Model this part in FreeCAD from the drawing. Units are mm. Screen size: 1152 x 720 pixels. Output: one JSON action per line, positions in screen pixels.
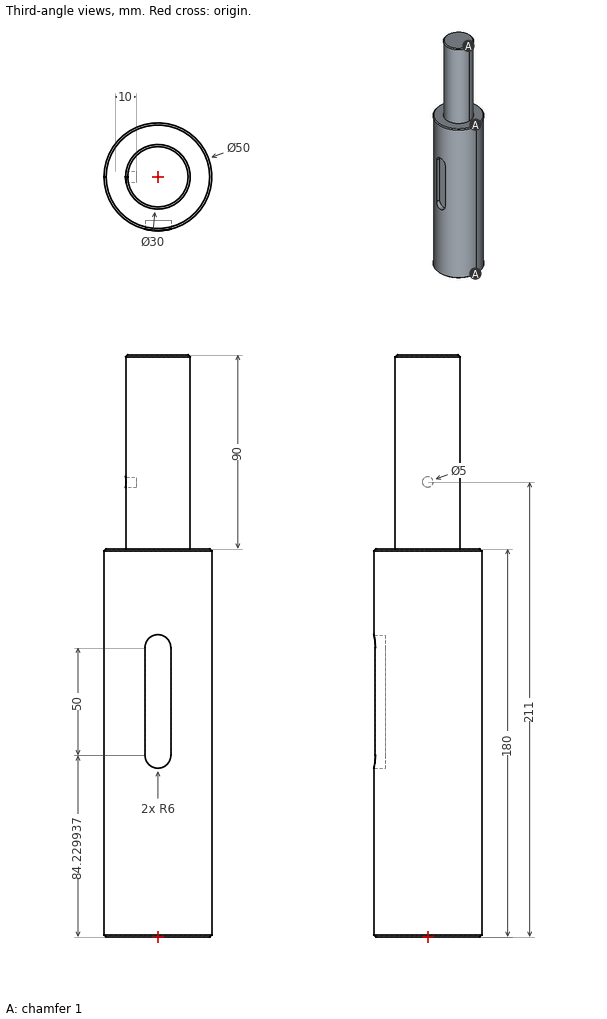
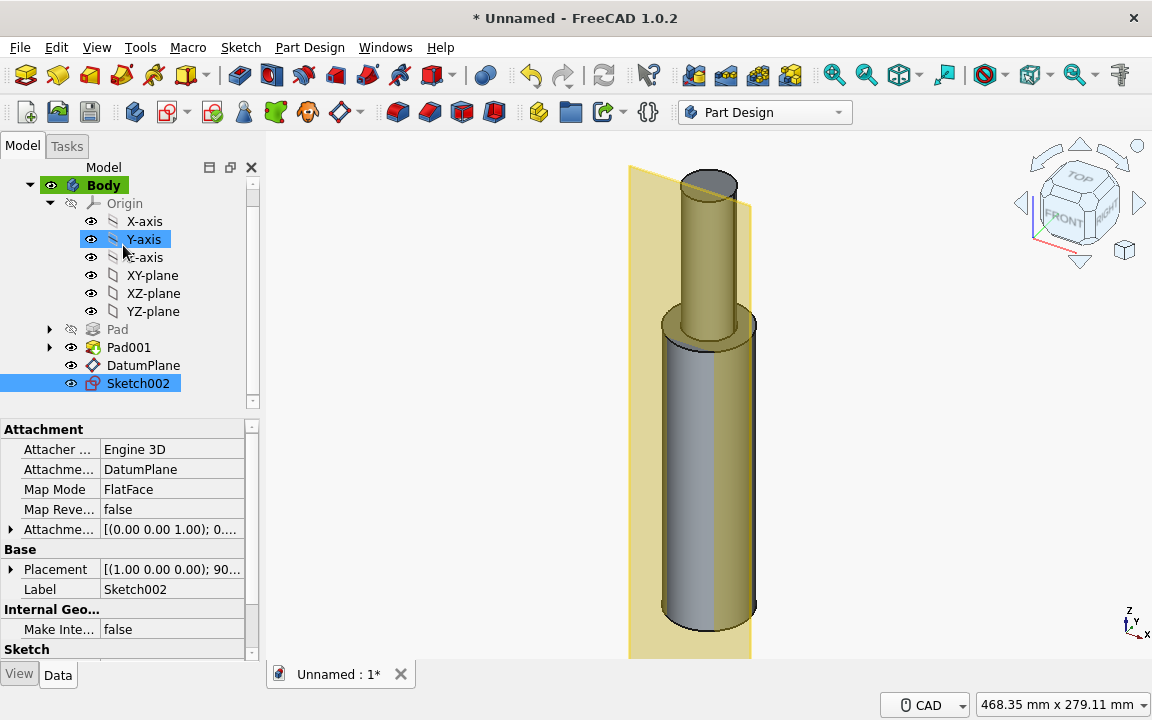
{"action": "left_click", "coordinate": [240, 76]}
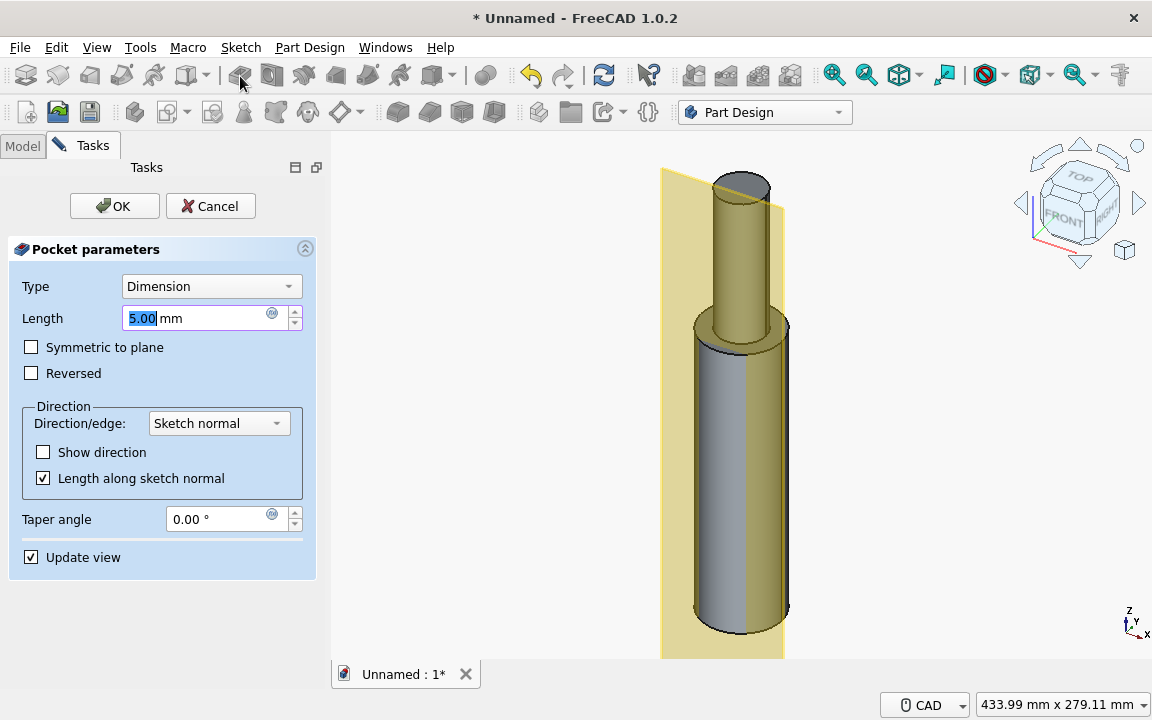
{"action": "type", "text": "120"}
{"action": "key", "text": "Tab"}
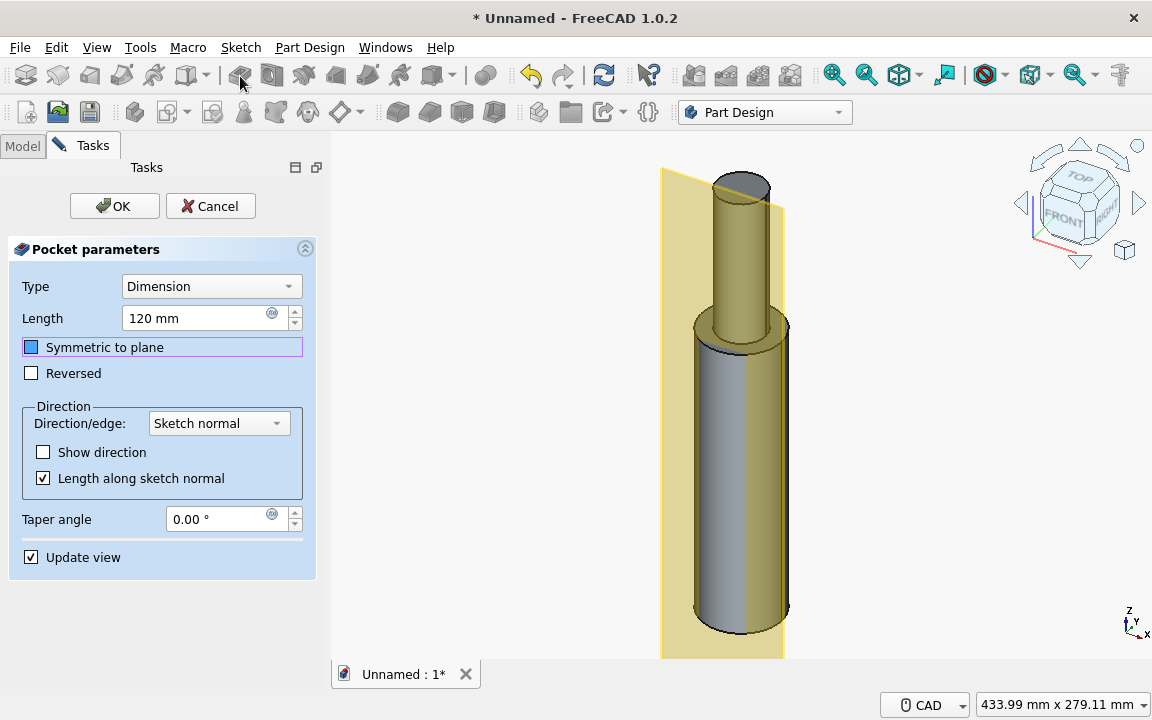
{"action": "left_click", "coordinate": [30, 373]}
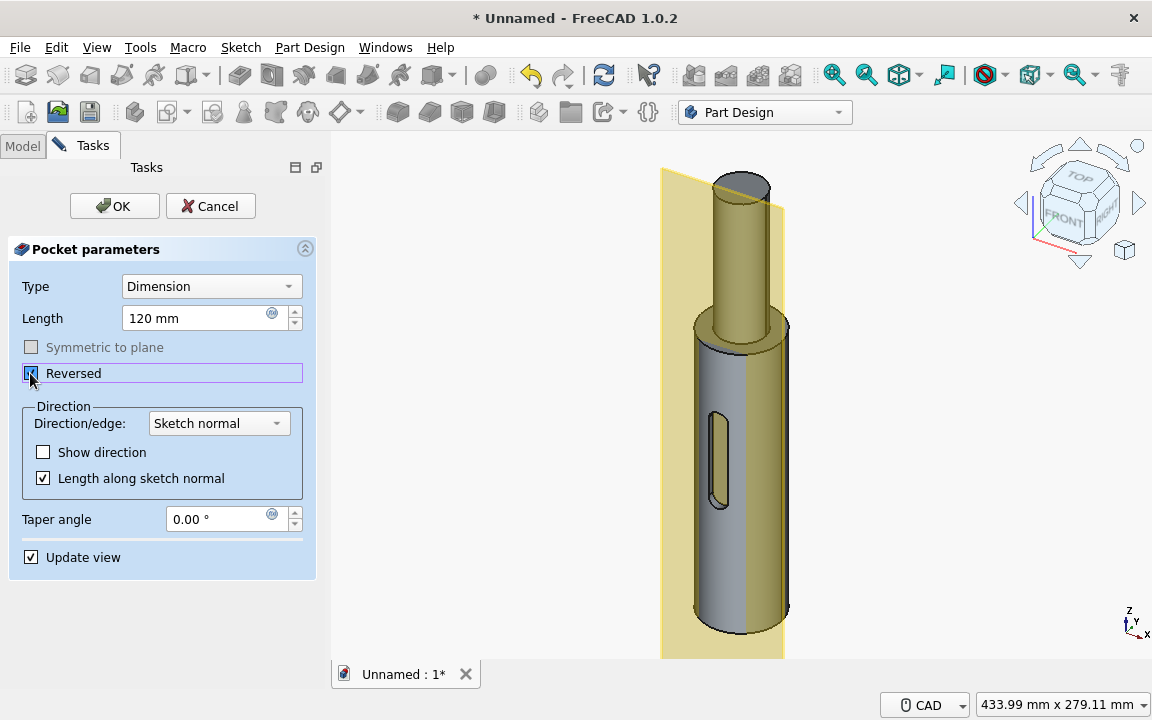
{"action": "left_click", "coordinate": [115, 206]}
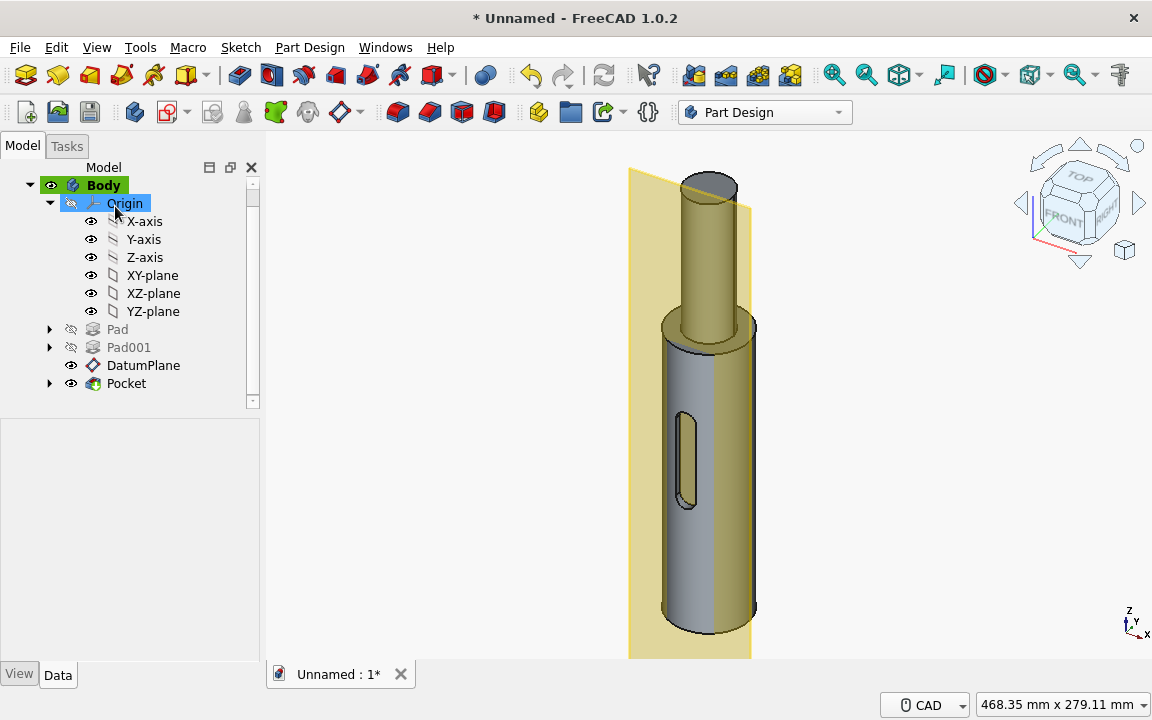
{"action": "left_click", "coordinate": [116, 365]}
{"action": "key", "text": "space"}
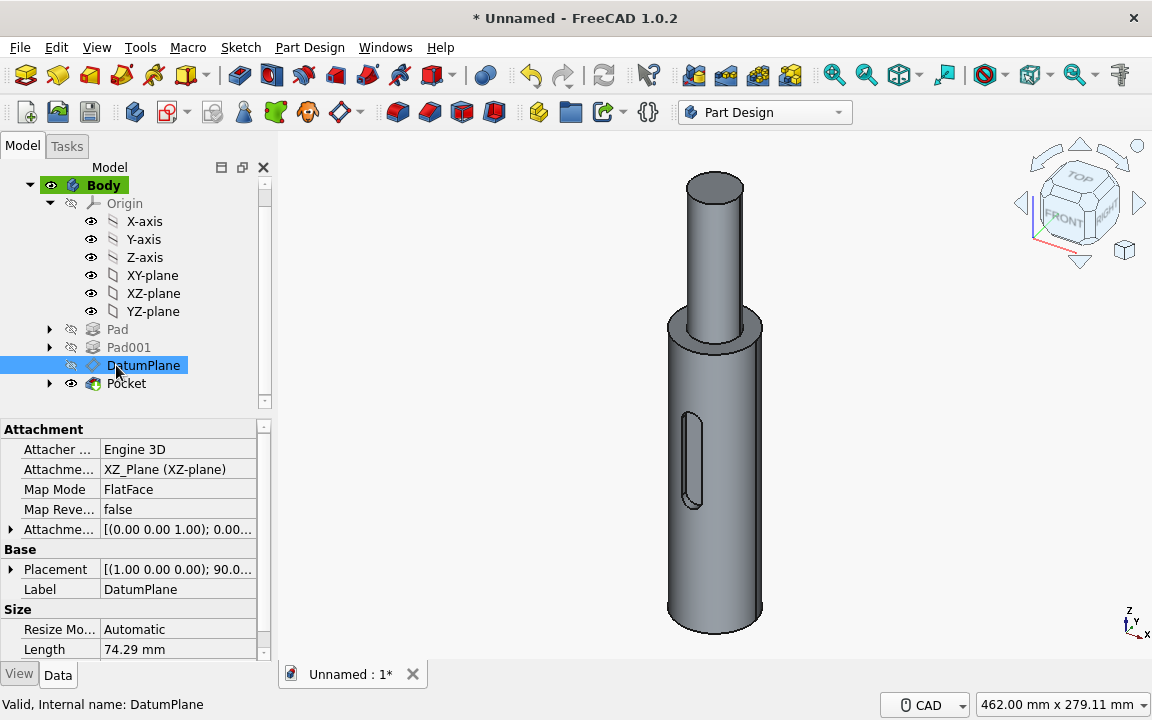
{"action": "left_click", "coordinate": [668, 330]}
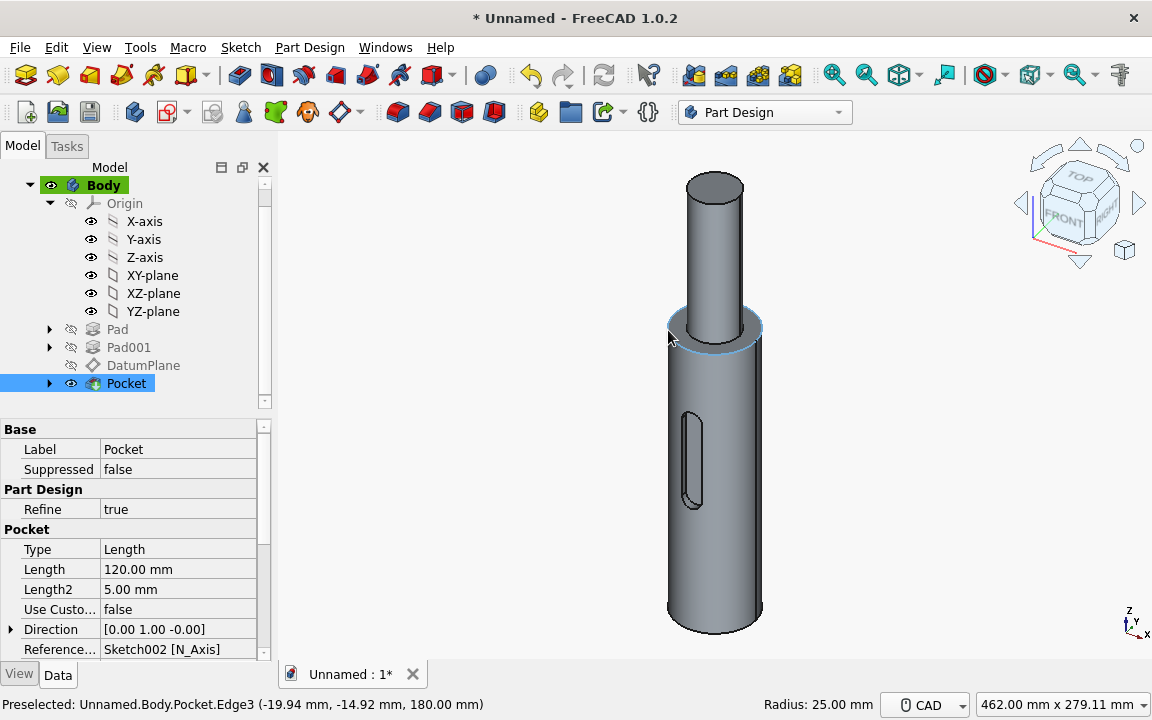
{"action": "left_click", "coordinate": [703, 172], "text": "ctrl"}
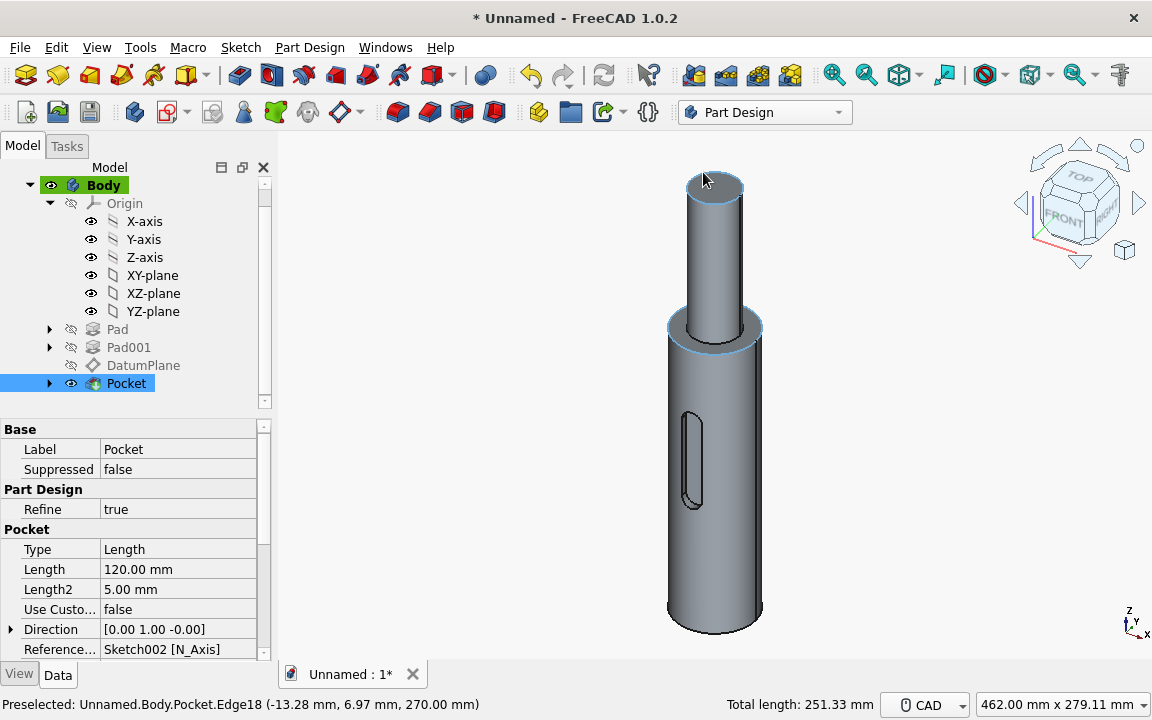
{"action": "key", "text": "0"}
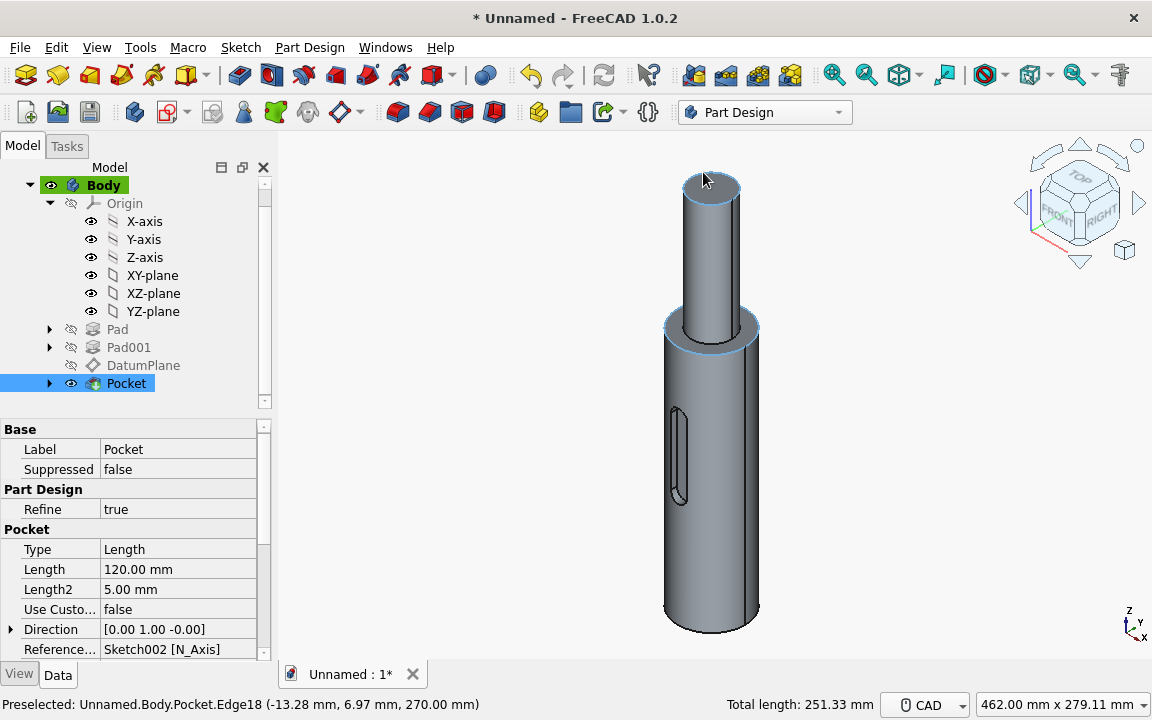
{"action": "key", "text": "2"}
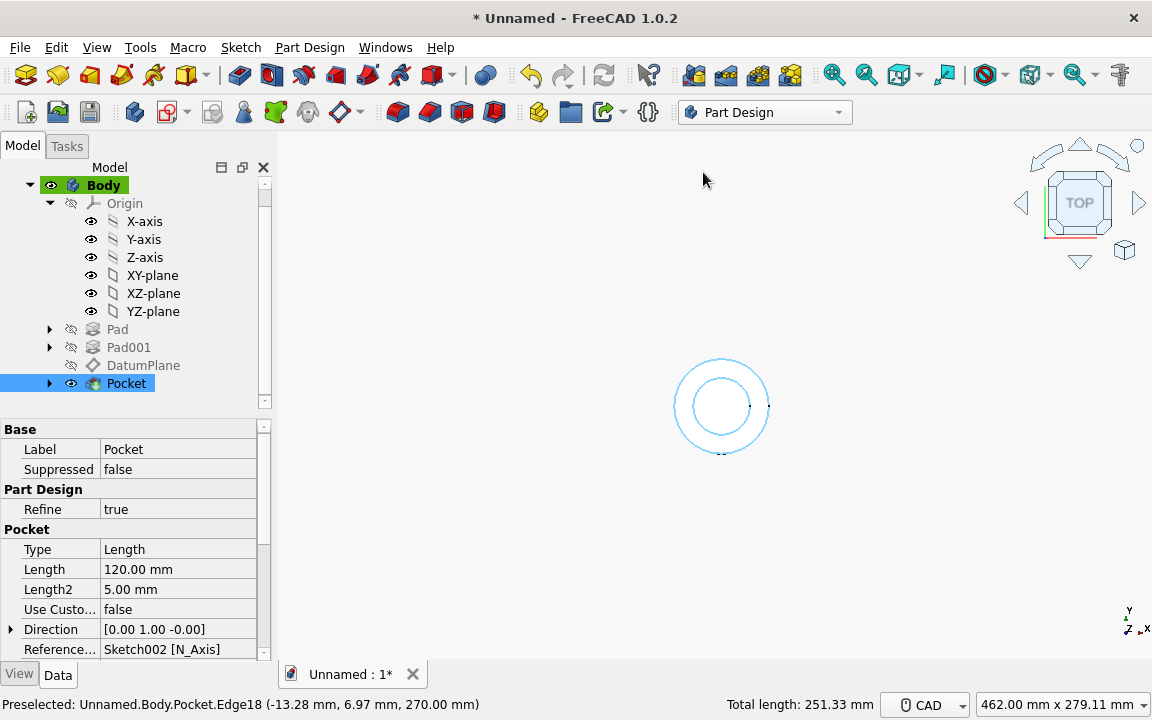
{"action": "left_click", "coordinate": [836, 76]}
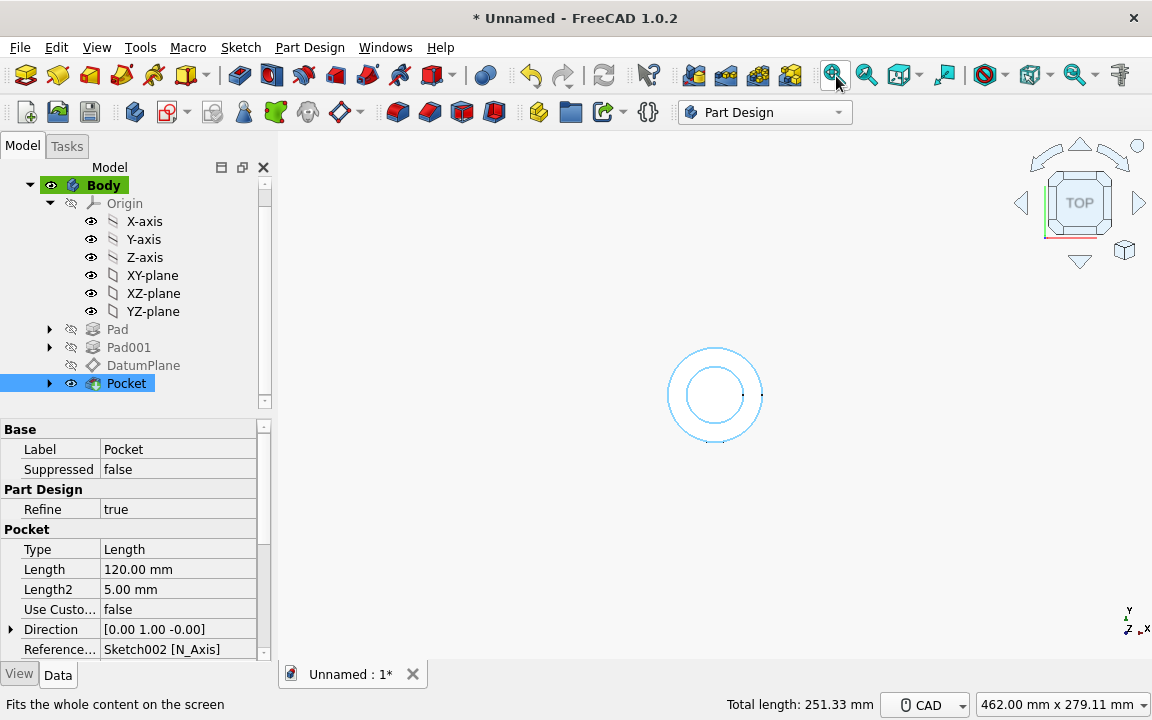
{"action": "key", "text": "1"}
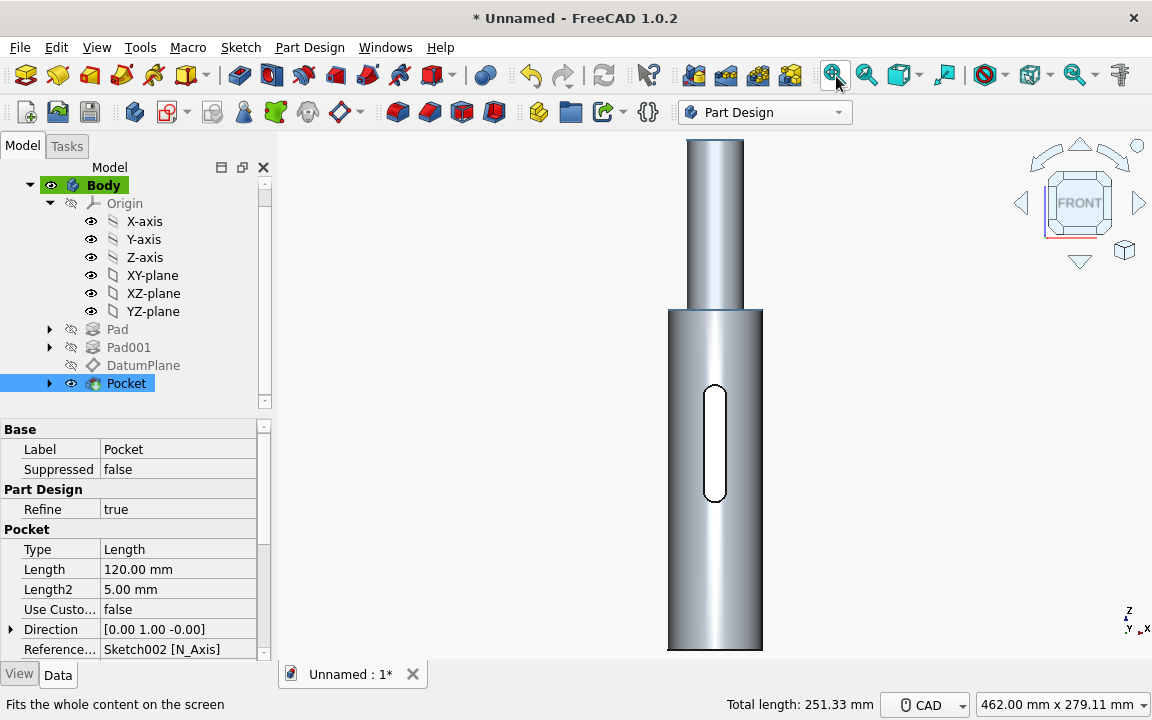
{"action": "key", "text": "3"}